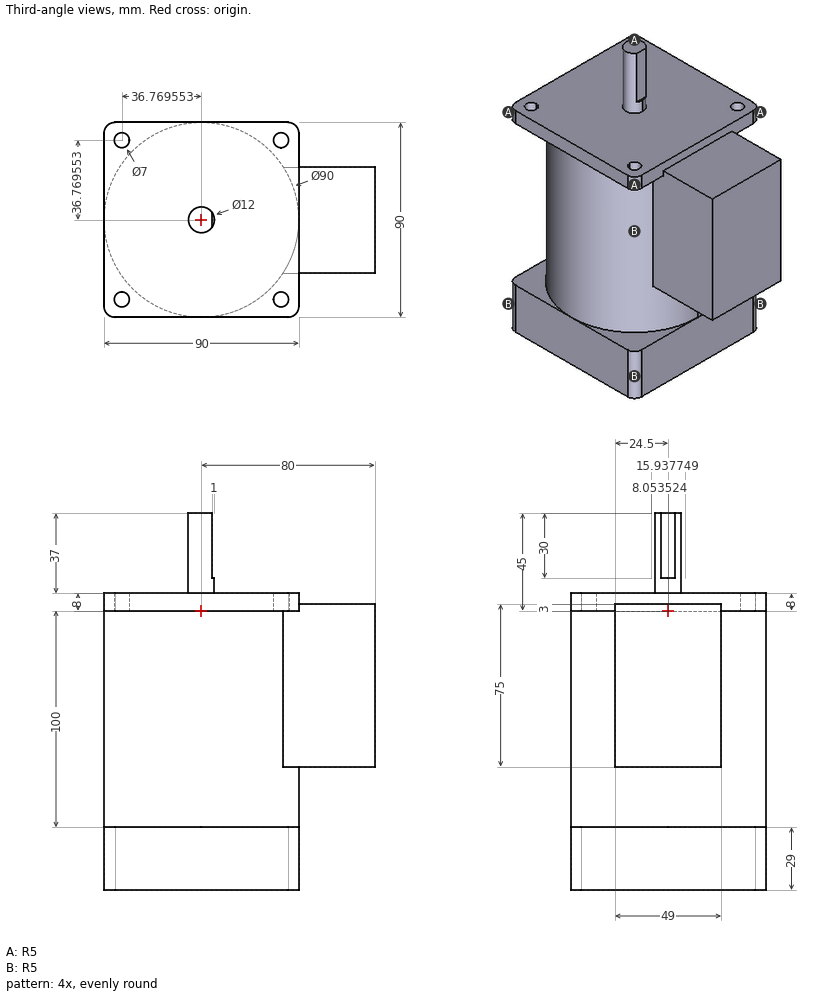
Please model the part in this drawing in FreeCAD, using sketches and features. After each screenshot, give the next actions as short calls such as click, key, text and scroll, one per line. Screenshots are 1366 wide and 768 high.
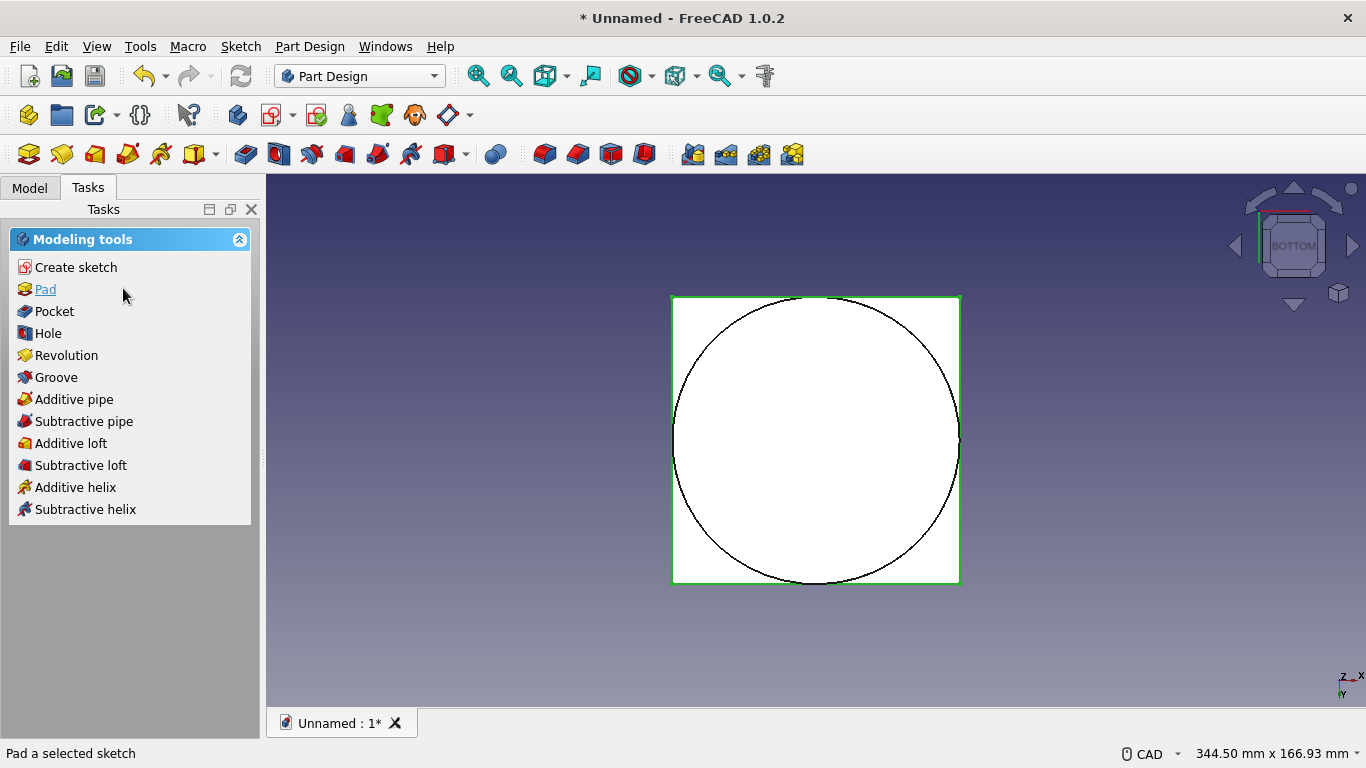
click(29, 154)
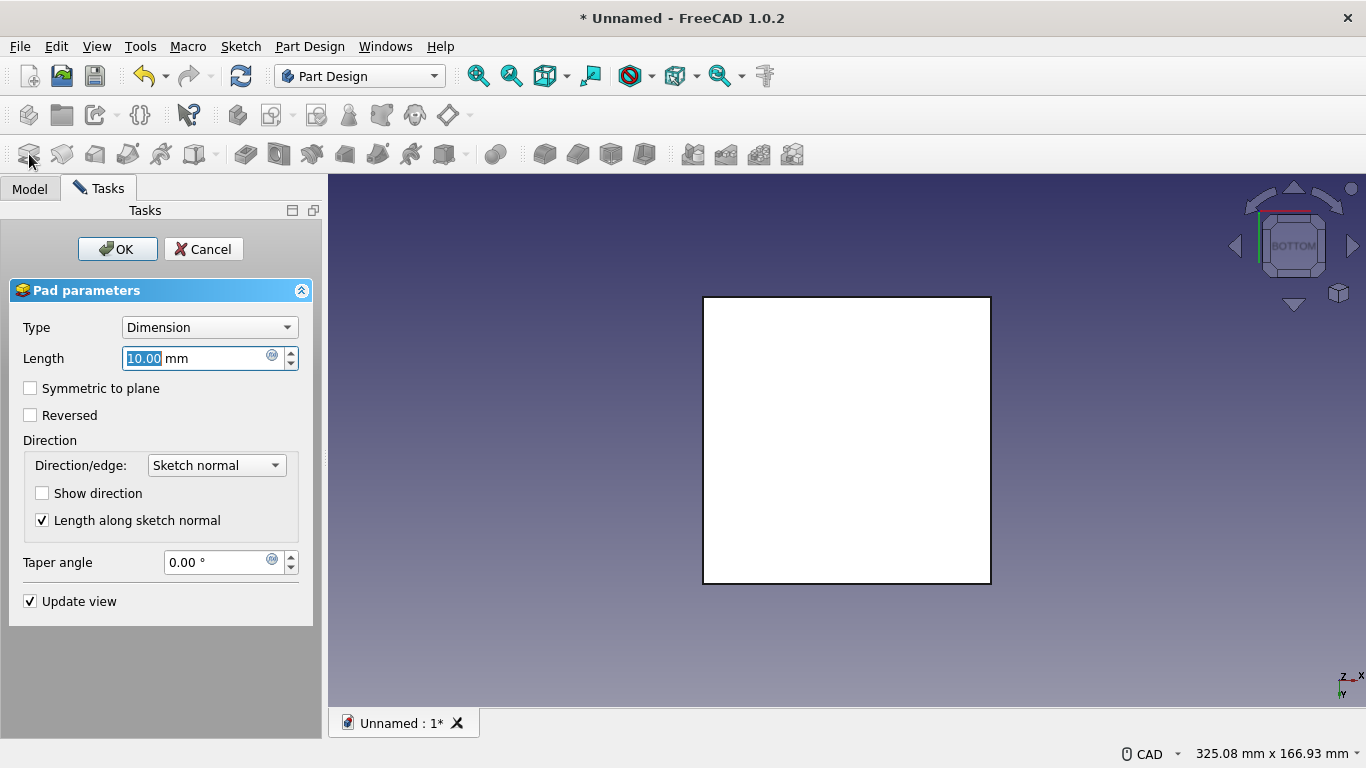
text(29)
key(Tab)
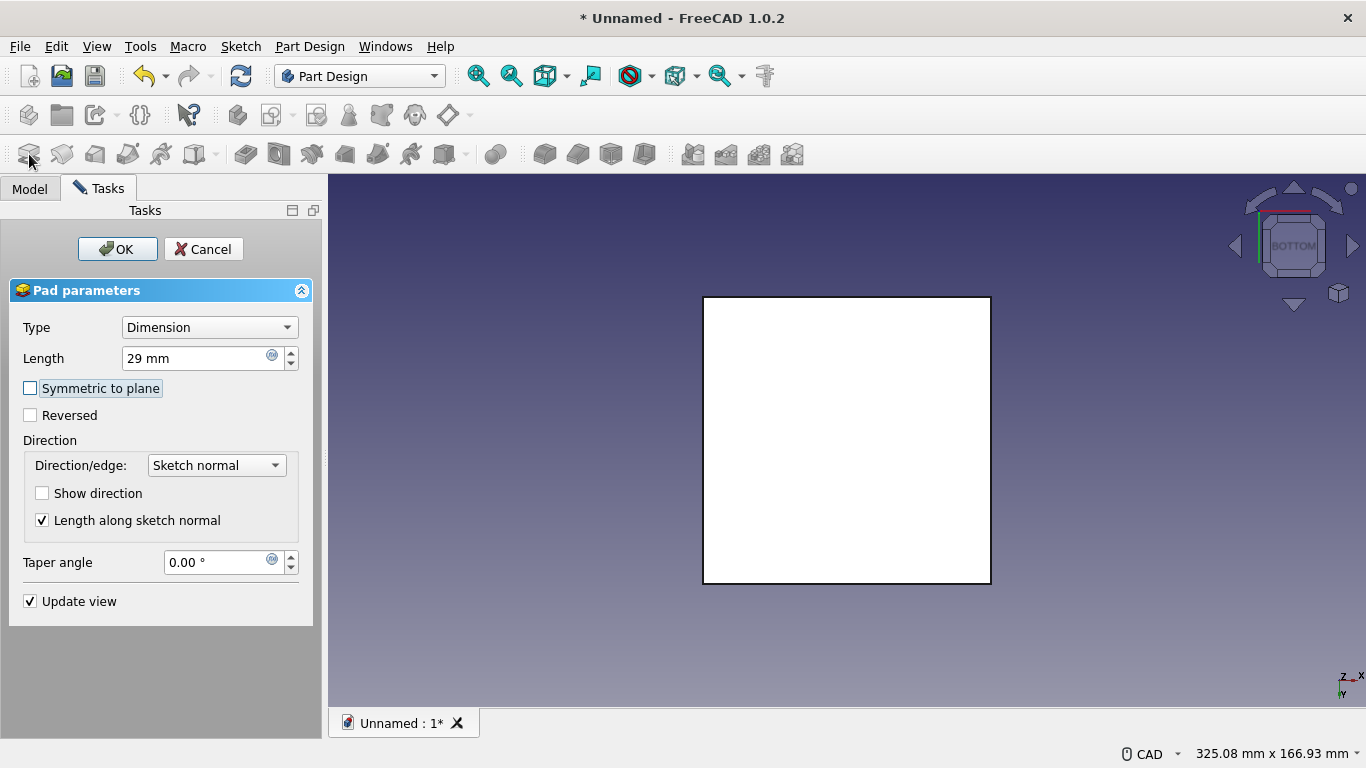
click(118, 249)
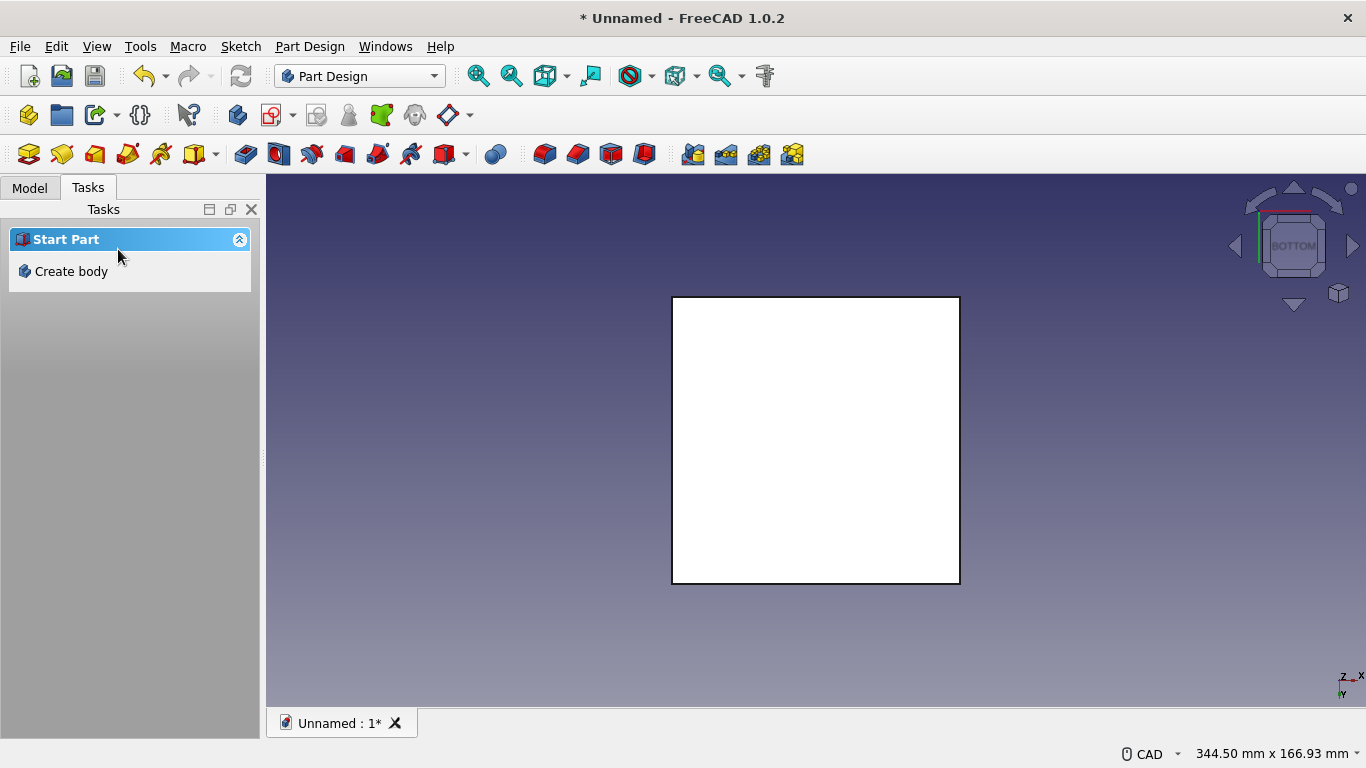
key(0)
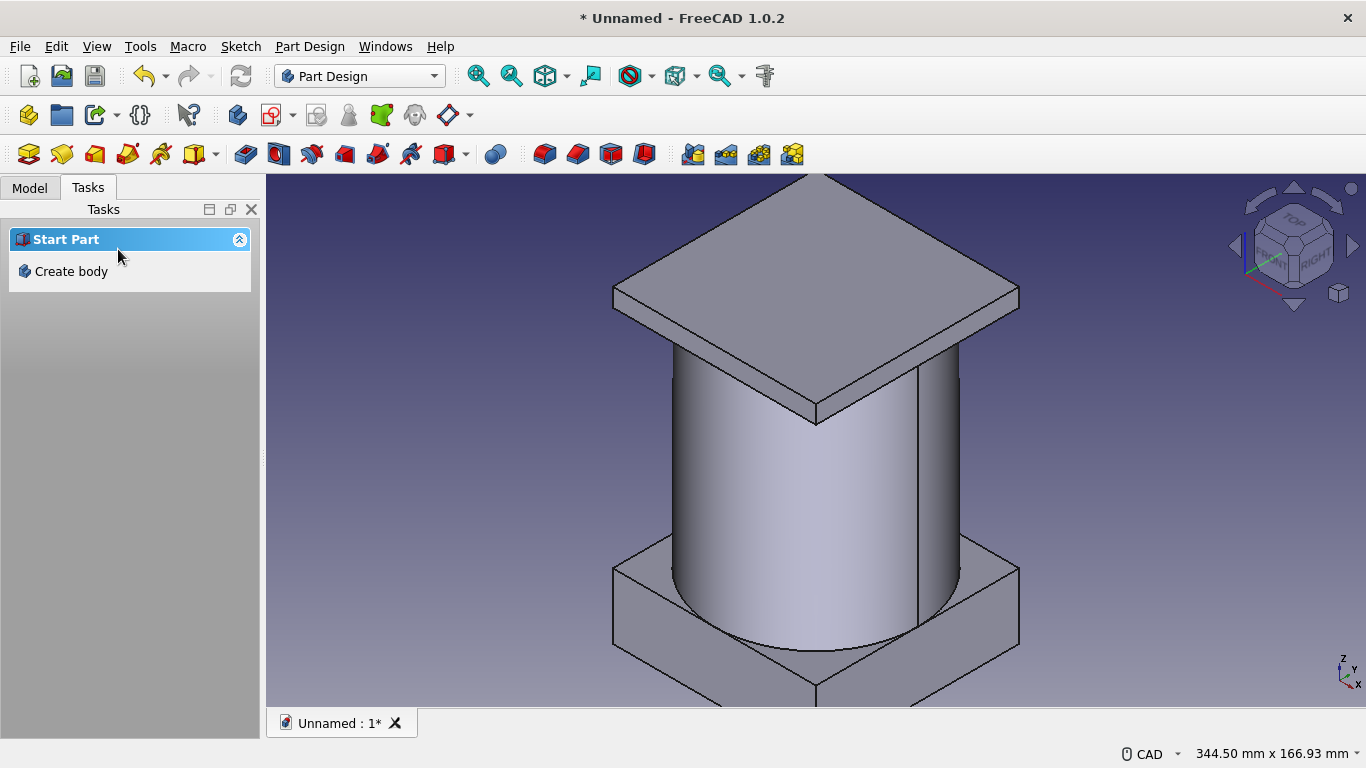
click(479, 76)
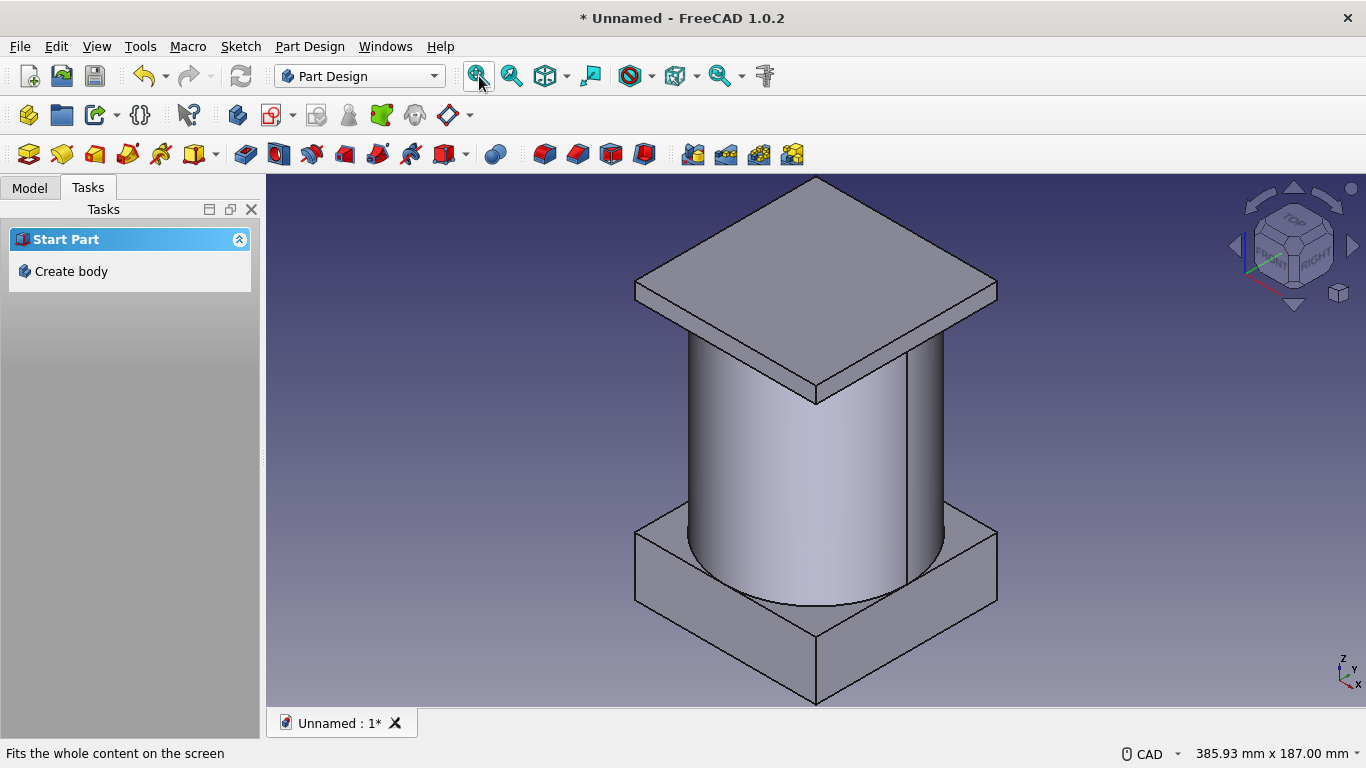
click(816, 280)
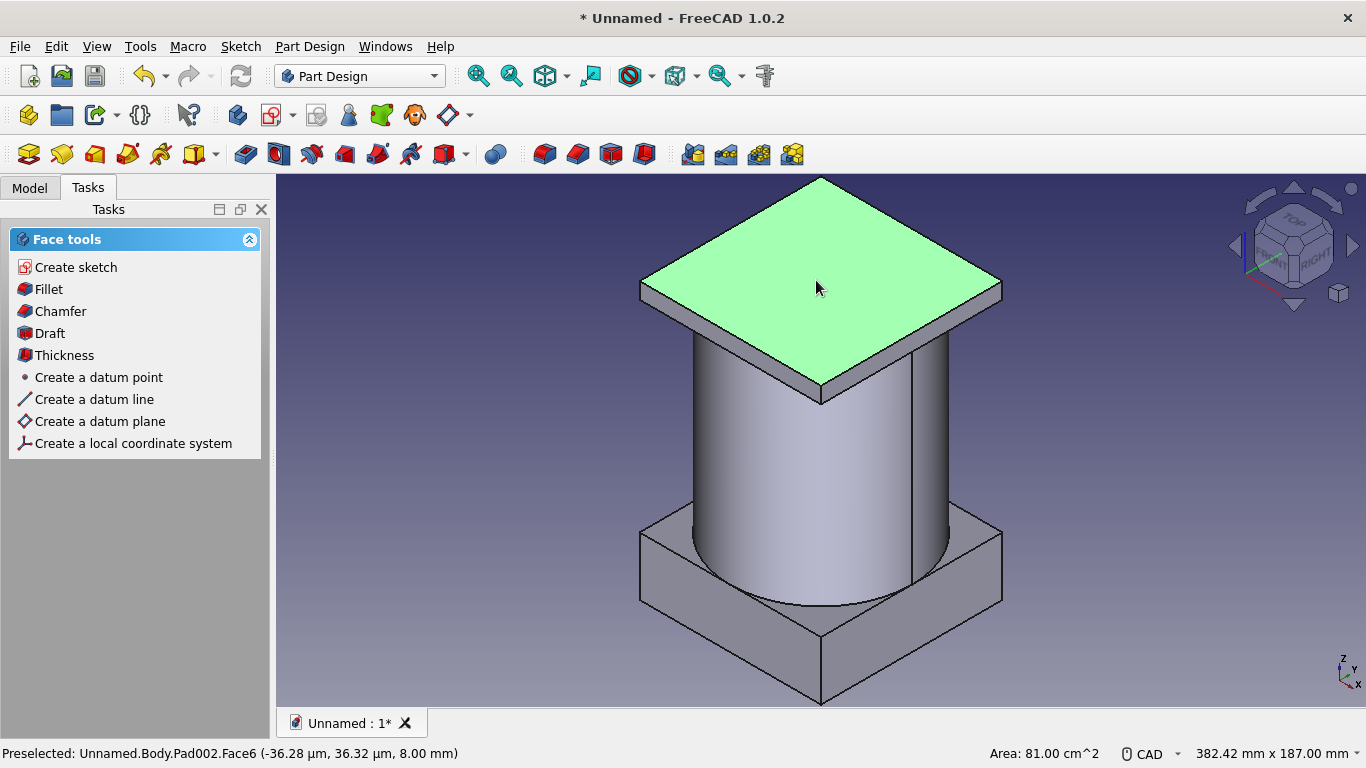
click(270, 116)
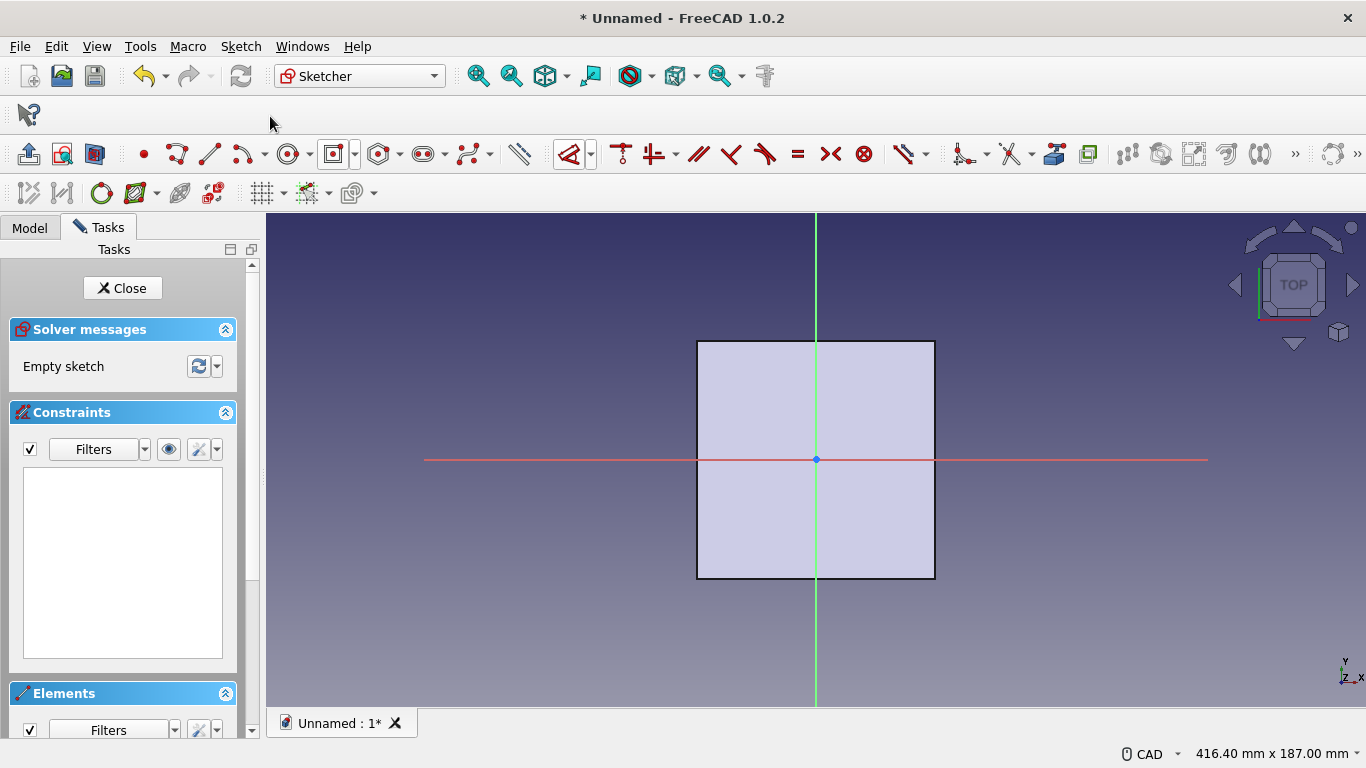
scroll(825, 460, up, 11)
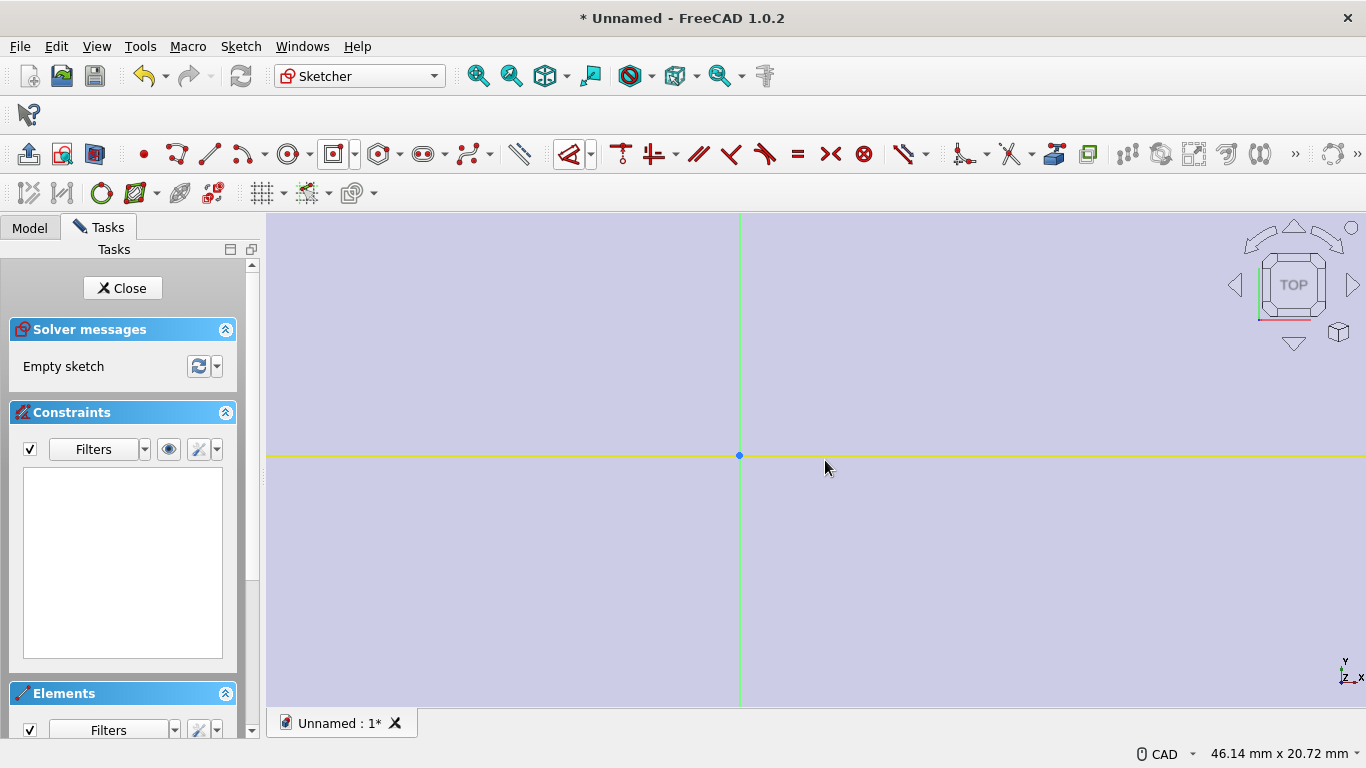
click(288, 154)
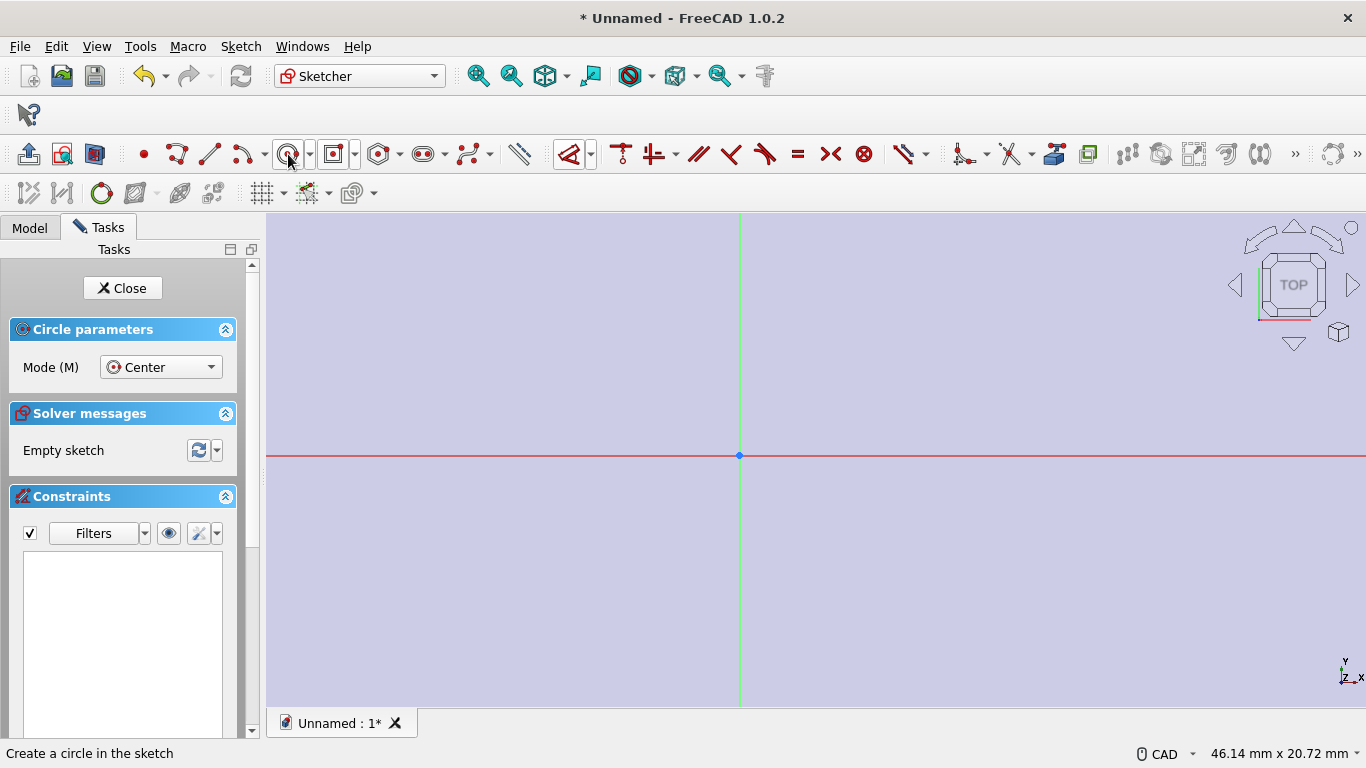
click(740, 456)
click(841, 355)
key(Escape)